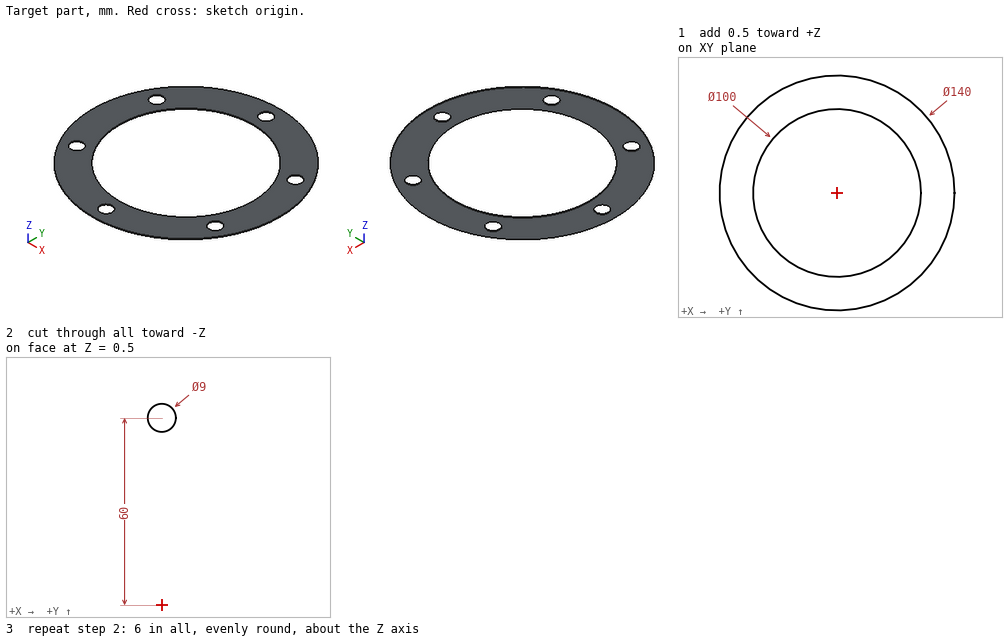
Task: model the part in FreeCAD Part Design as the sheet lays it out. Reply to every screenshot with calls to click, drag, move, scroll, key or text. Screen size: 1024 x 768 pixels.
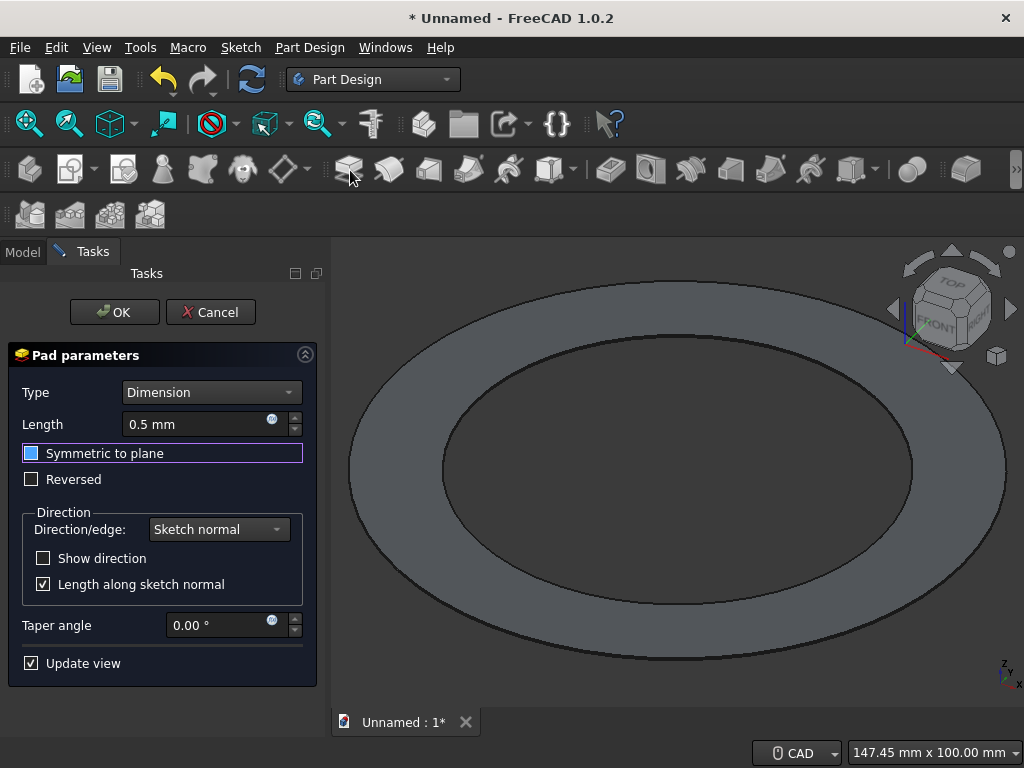
click(115, 312)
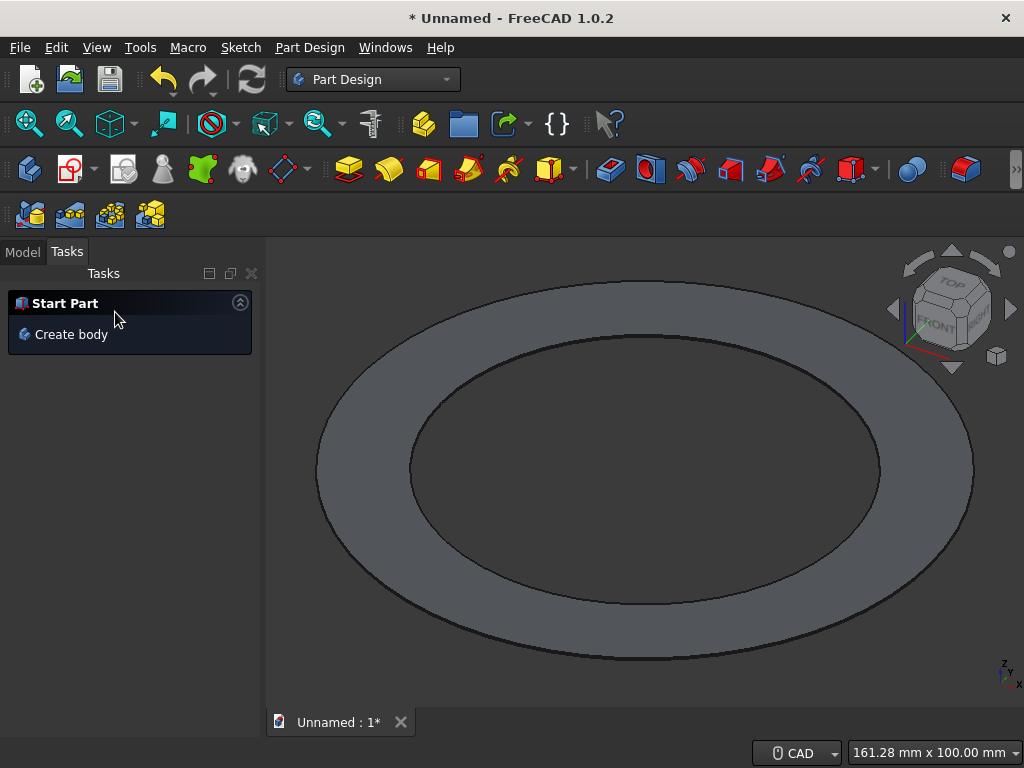
click(30, 124)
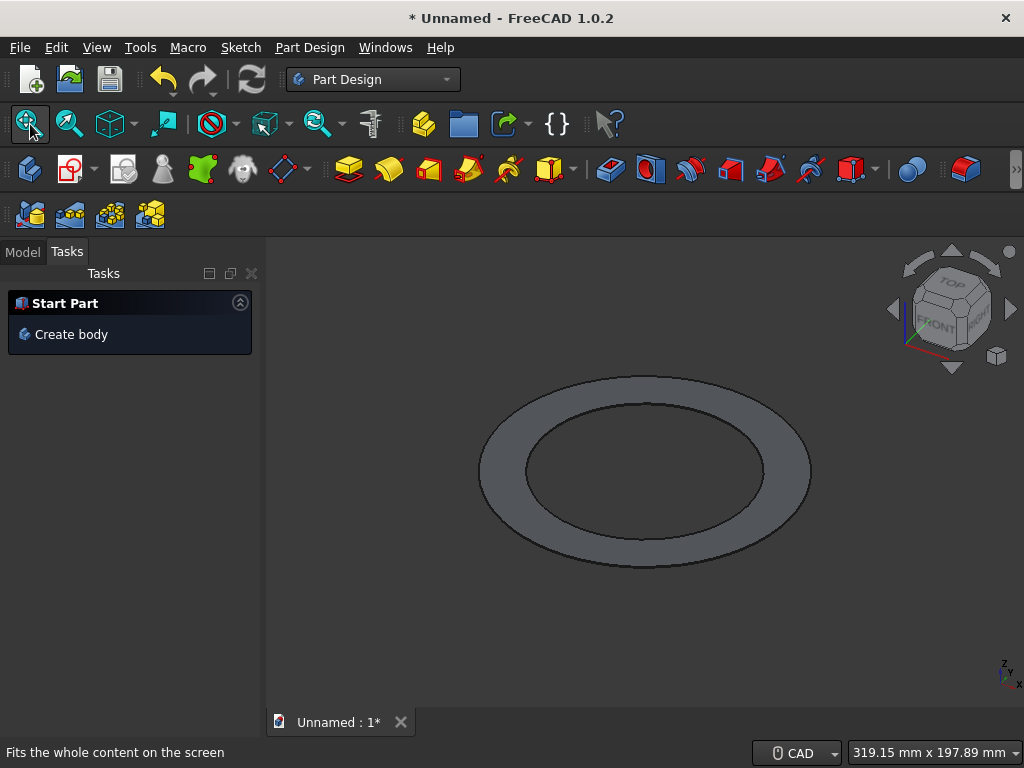
click(768, 511)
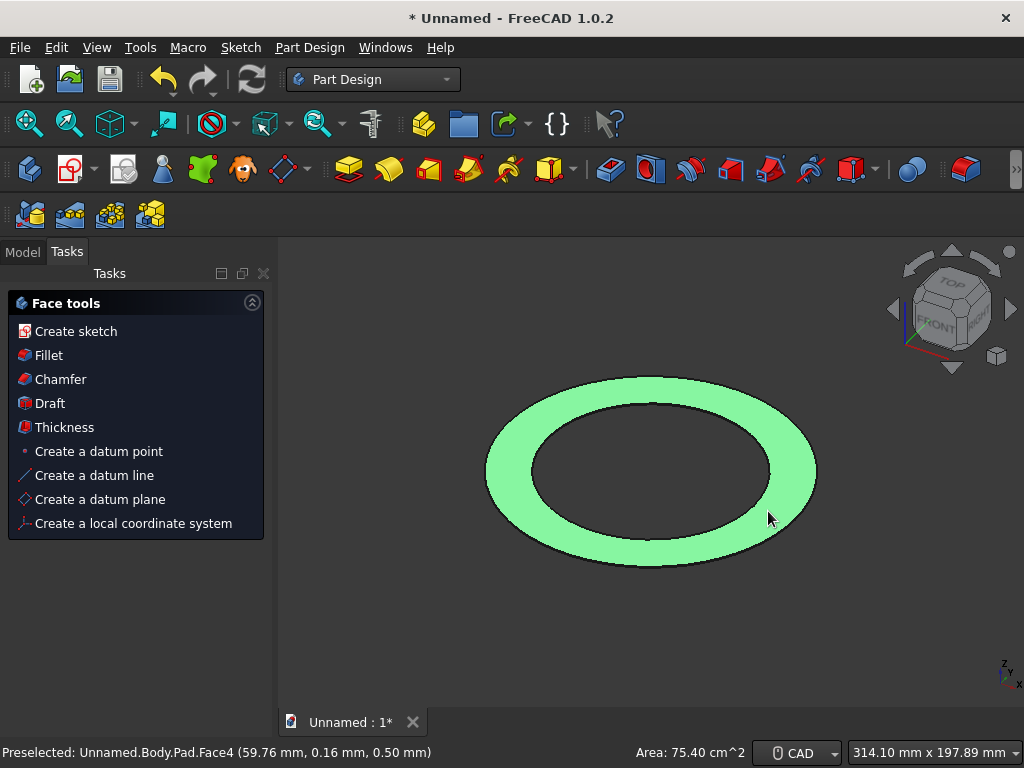
click(70, 170)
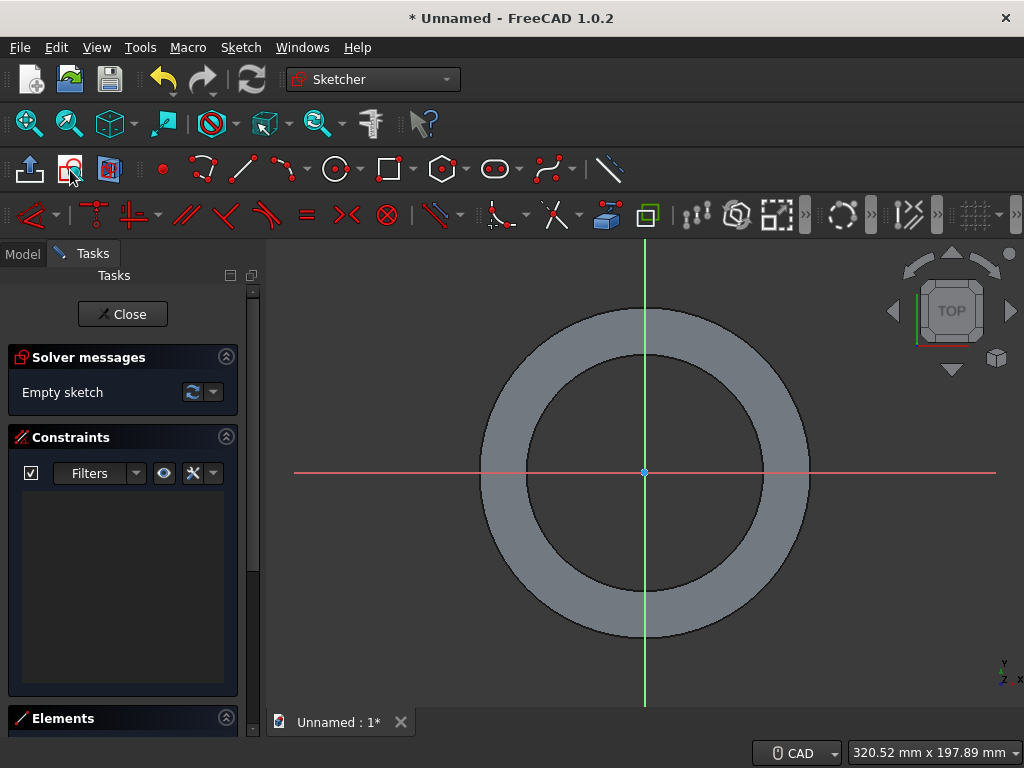
scroll(650, 320, up, 13)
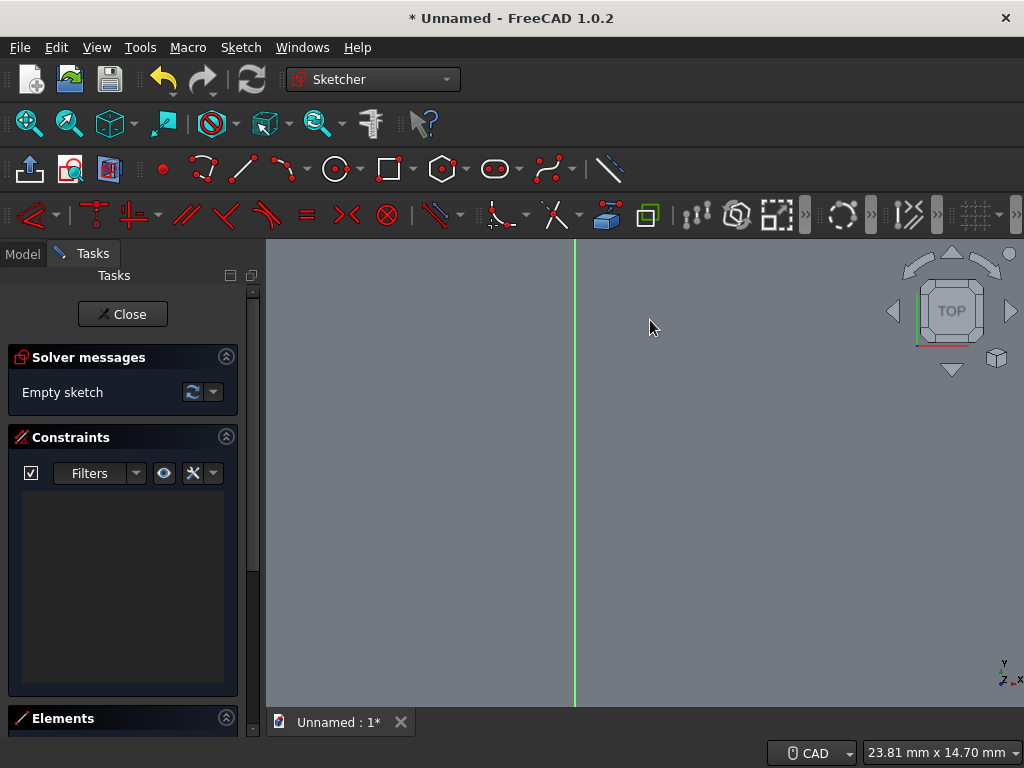
click(336, 170)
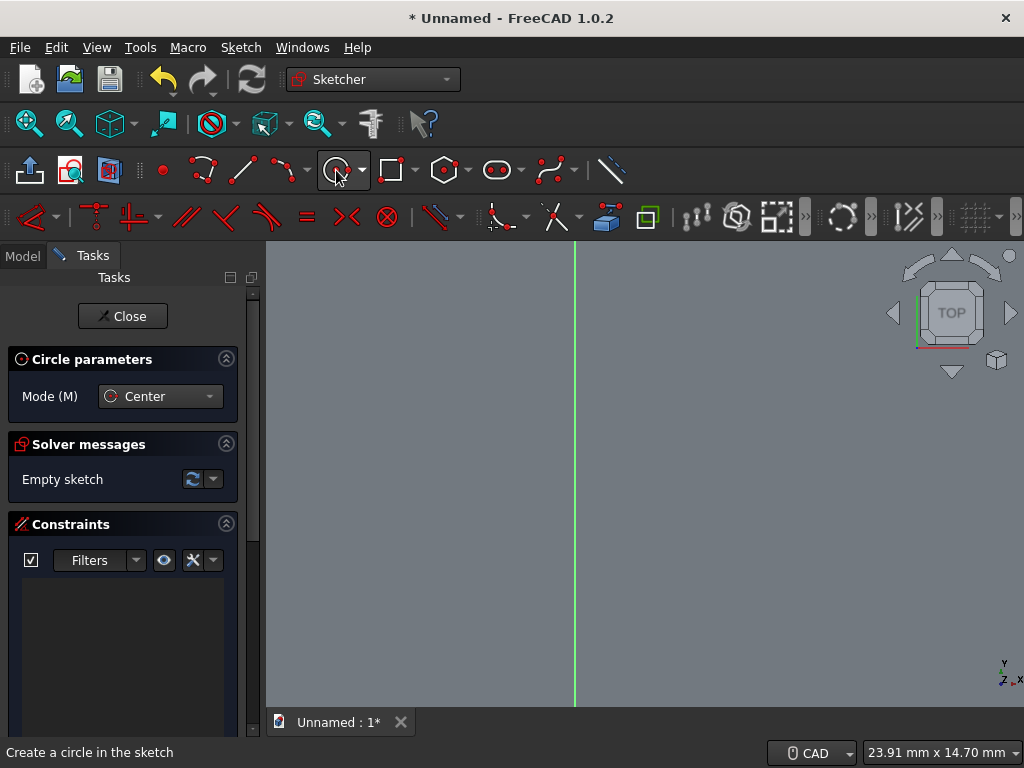
click(575, 468)
move(676, 367)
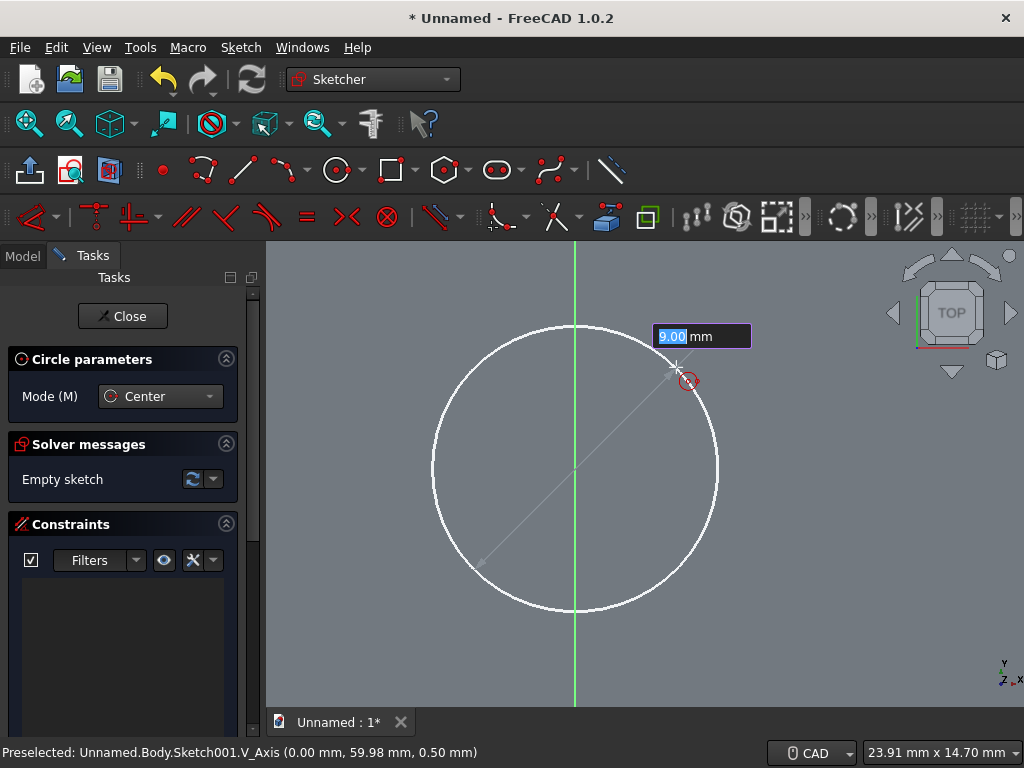
text(9)
key(Return)
key(Escape)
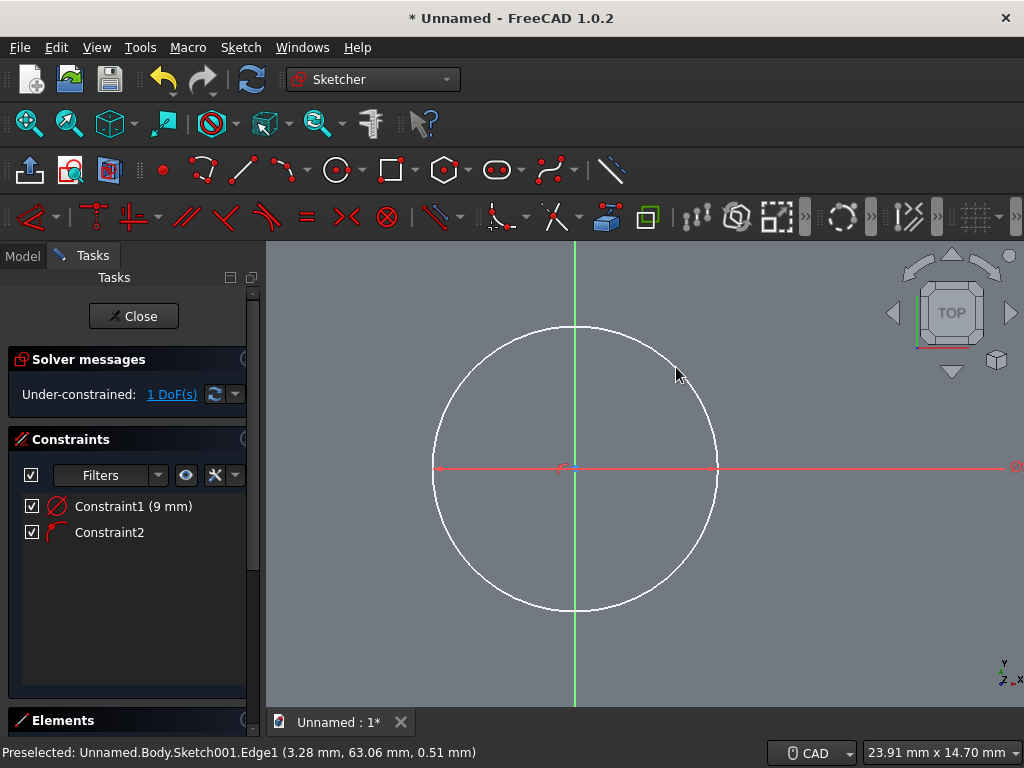
click(32, 218)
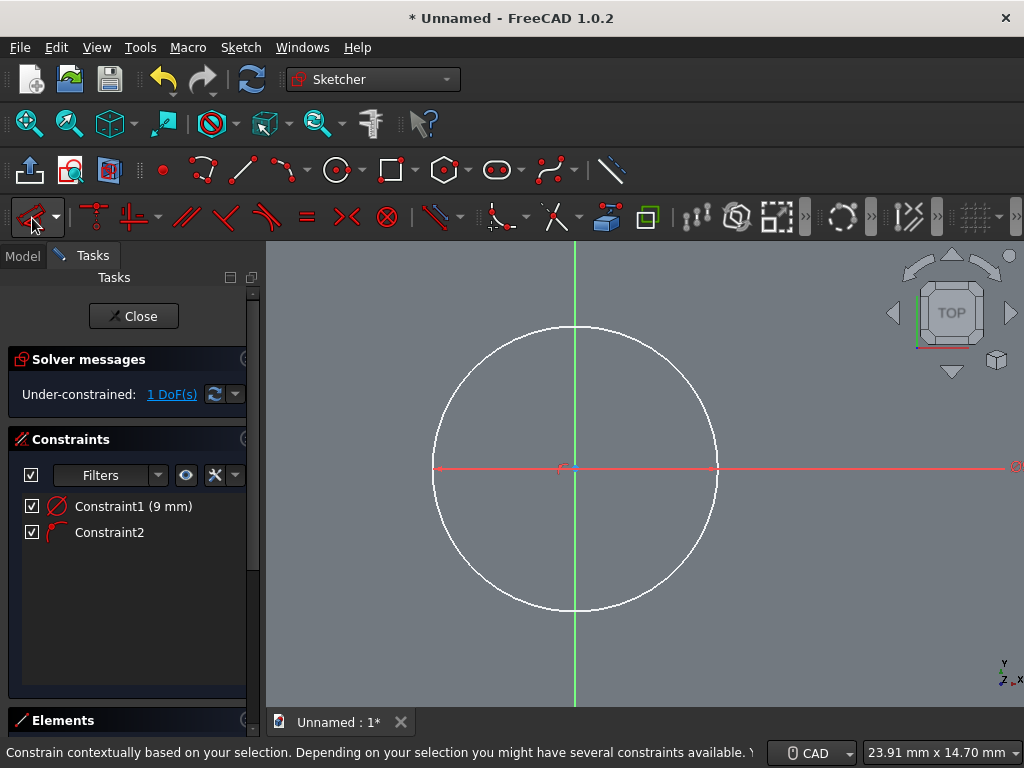
click(575, 469)
click(609, 574)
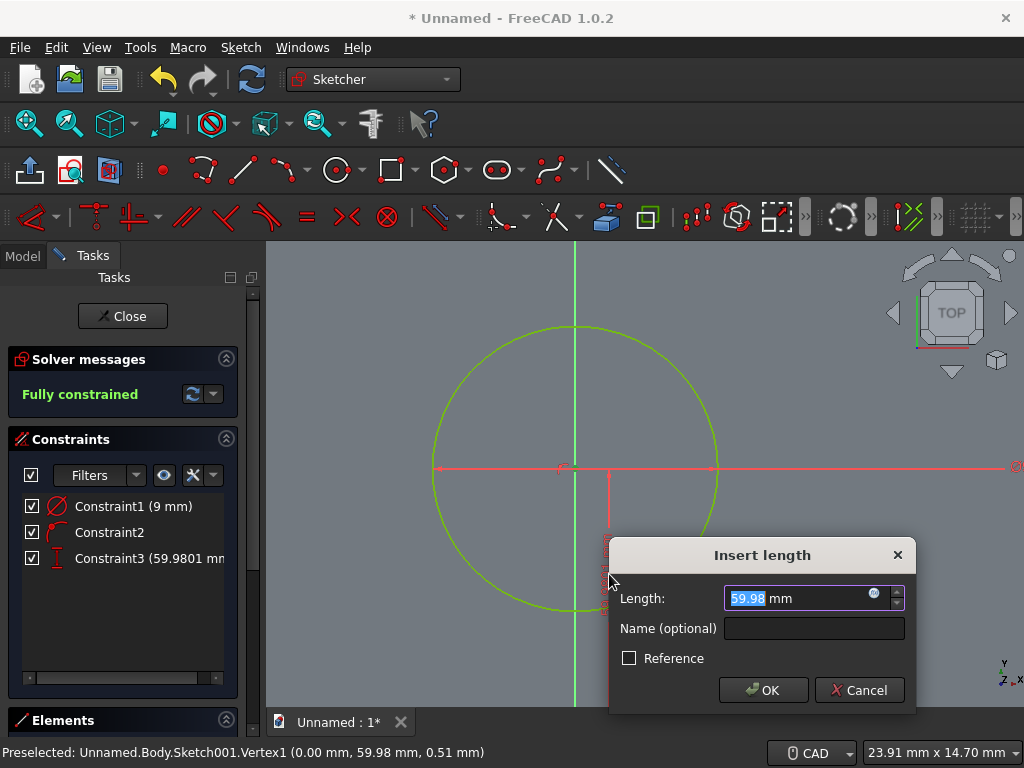
text(60)
key(Return)
key(Escape)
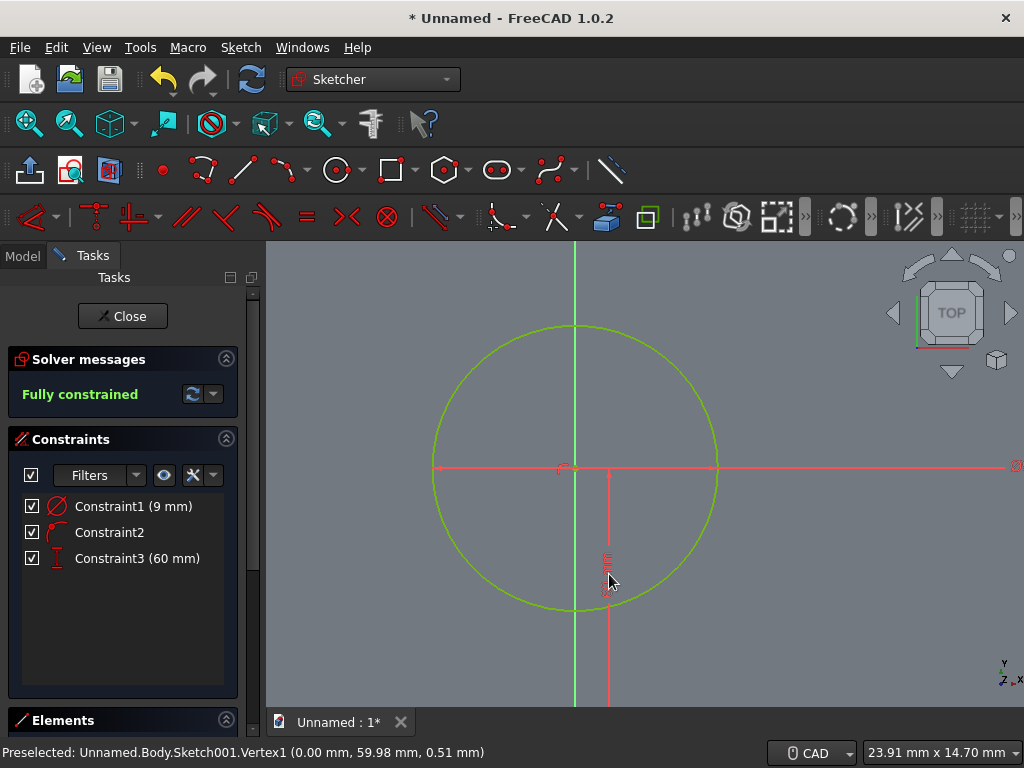
click(123, 316)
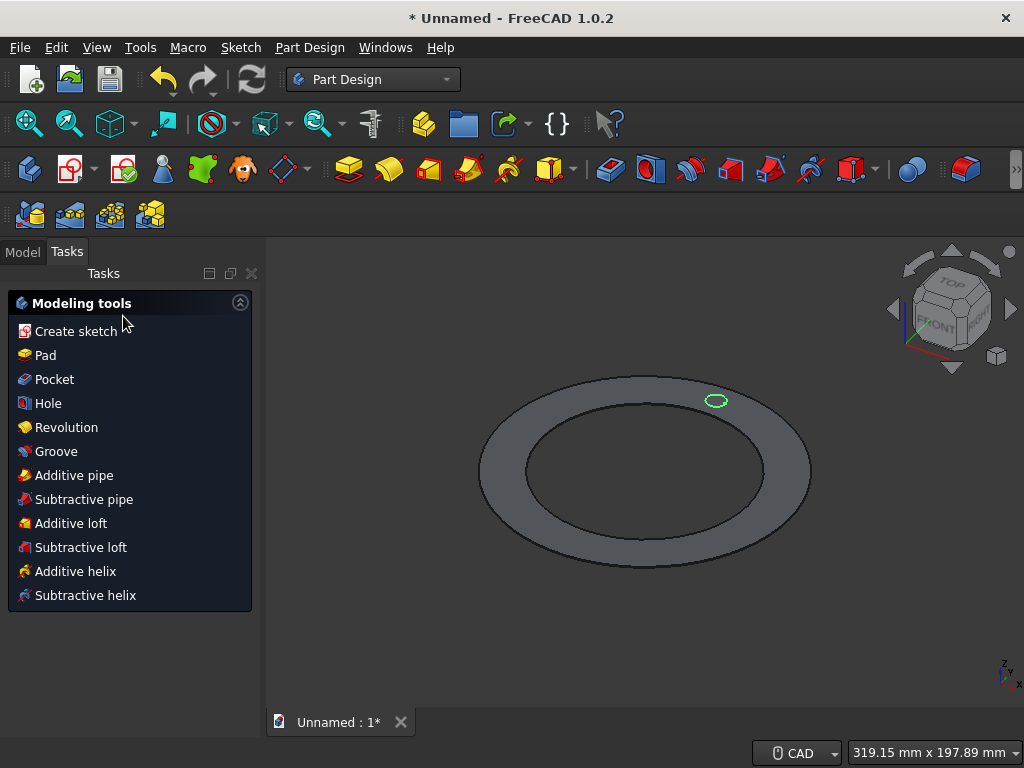
click(612, 170)